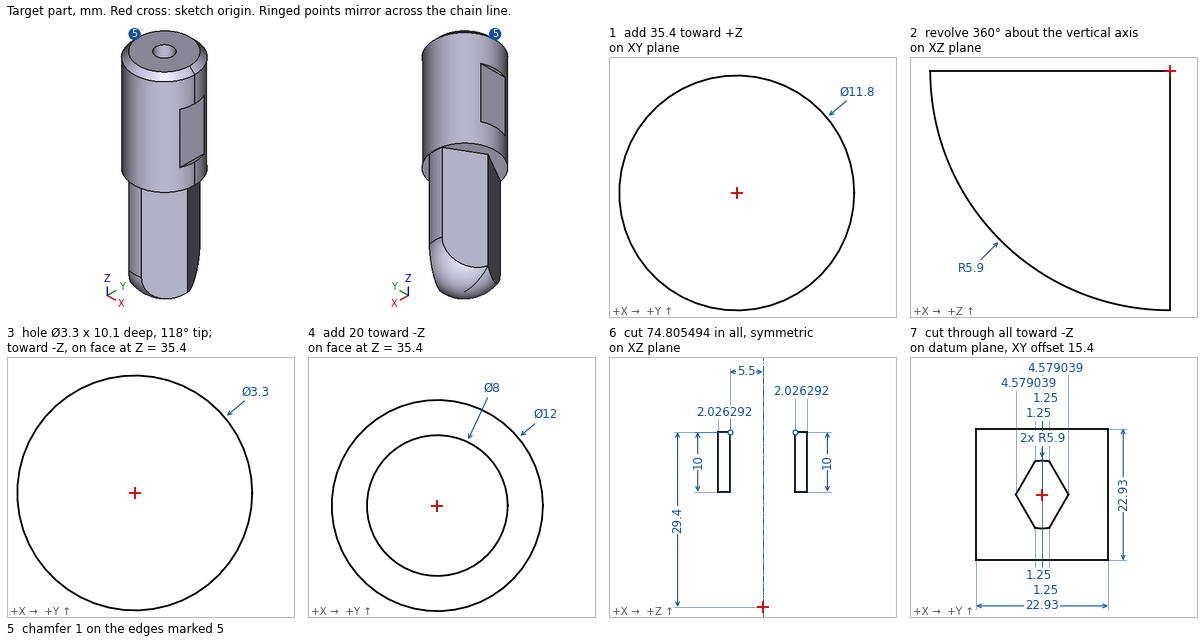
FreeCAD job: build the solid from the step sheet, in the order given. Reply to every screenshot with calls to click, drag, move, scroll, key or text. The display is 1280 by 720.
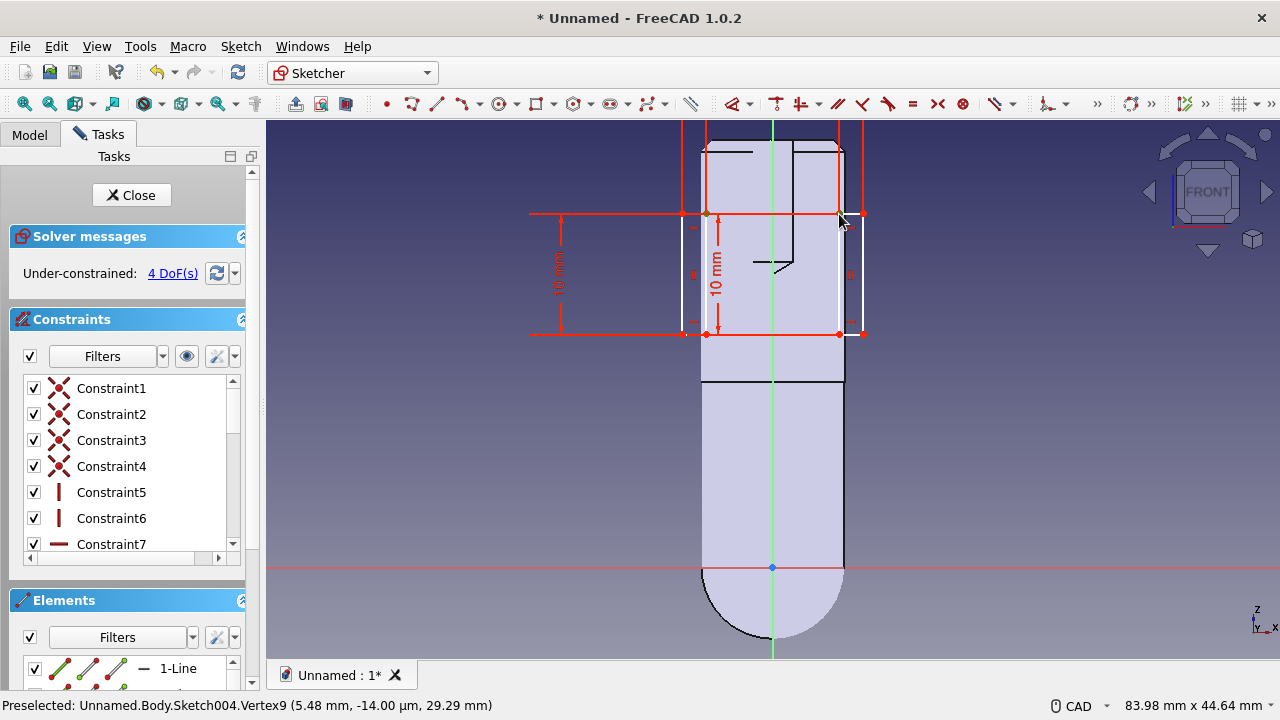
click(773, 528)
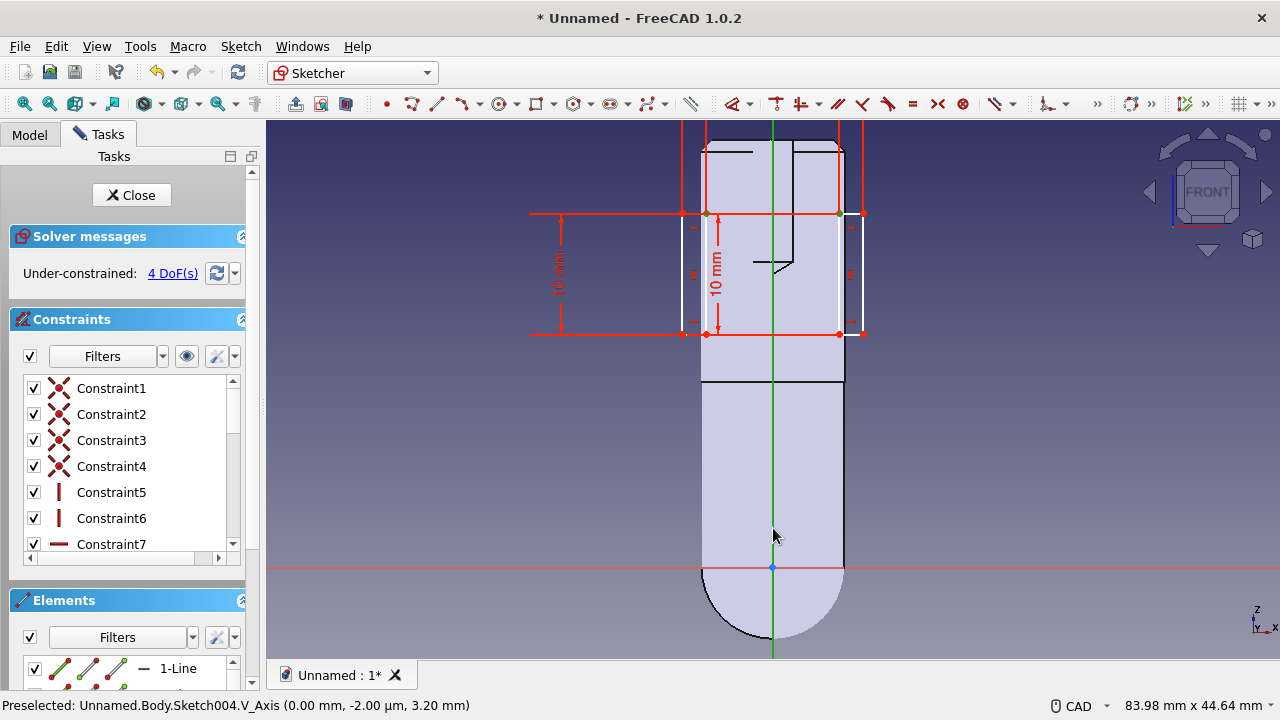
click(938, 104)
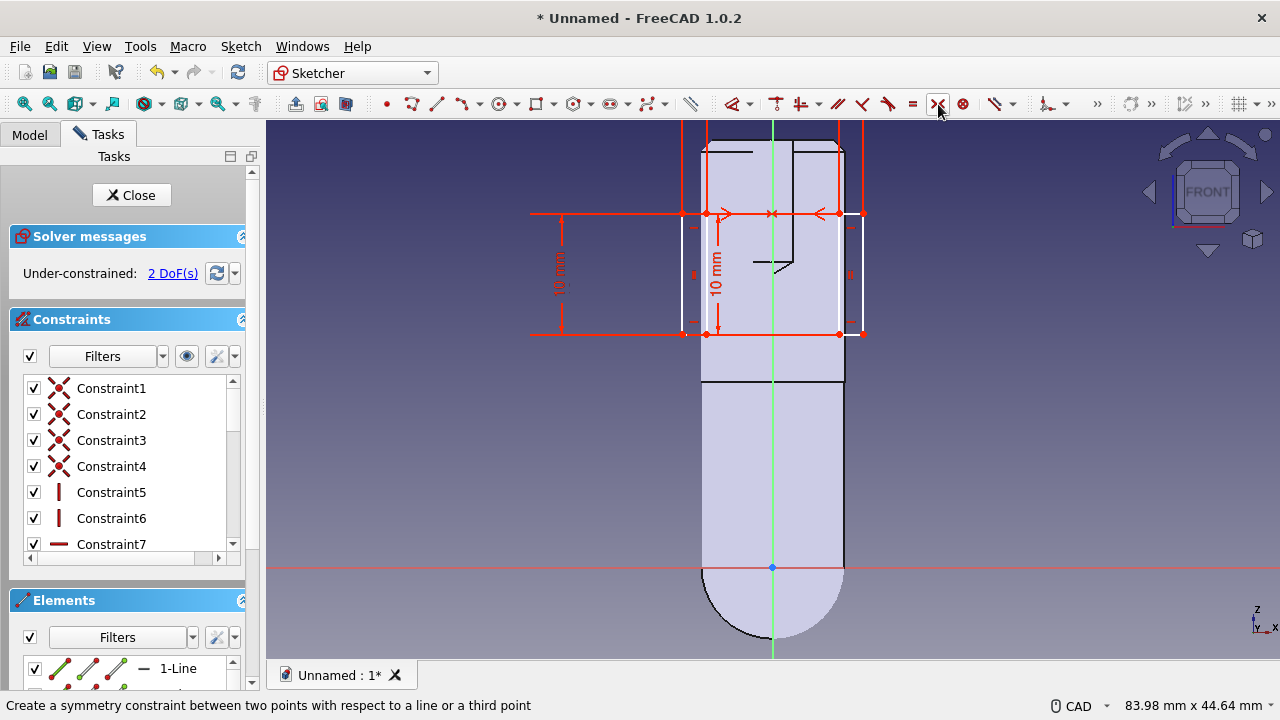
key(d)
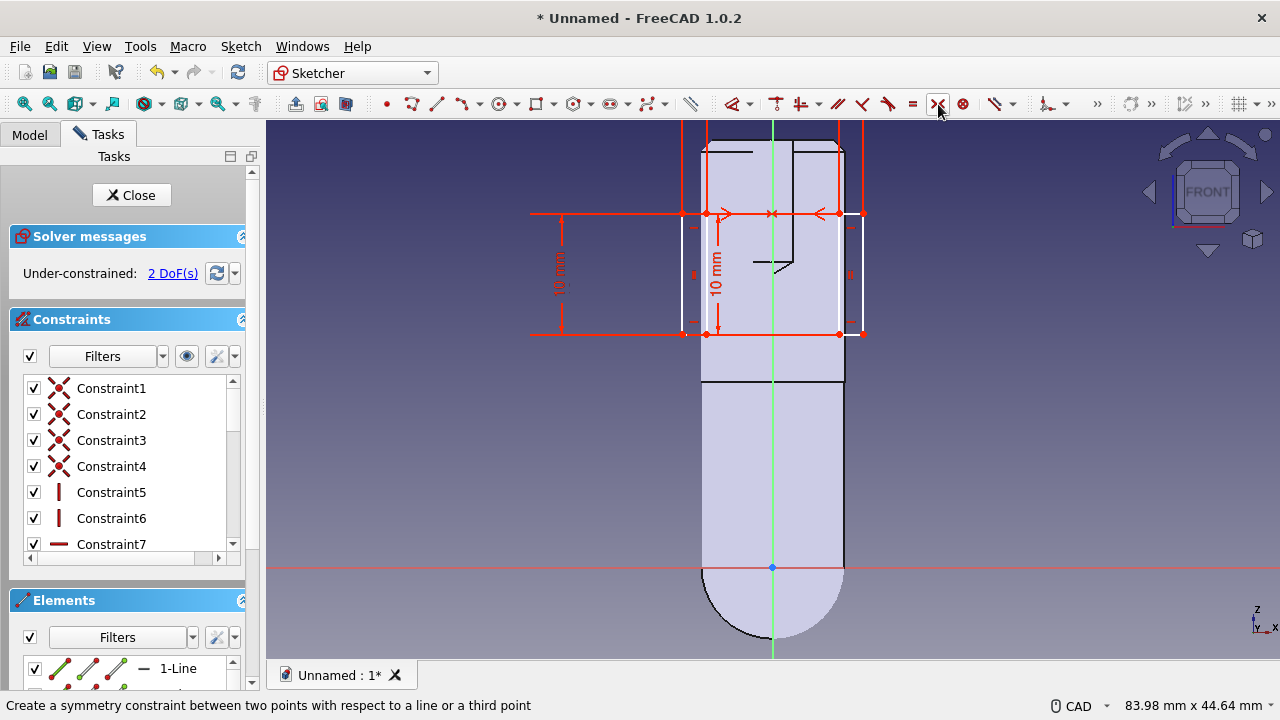
click(707, 335)
click(740, 602)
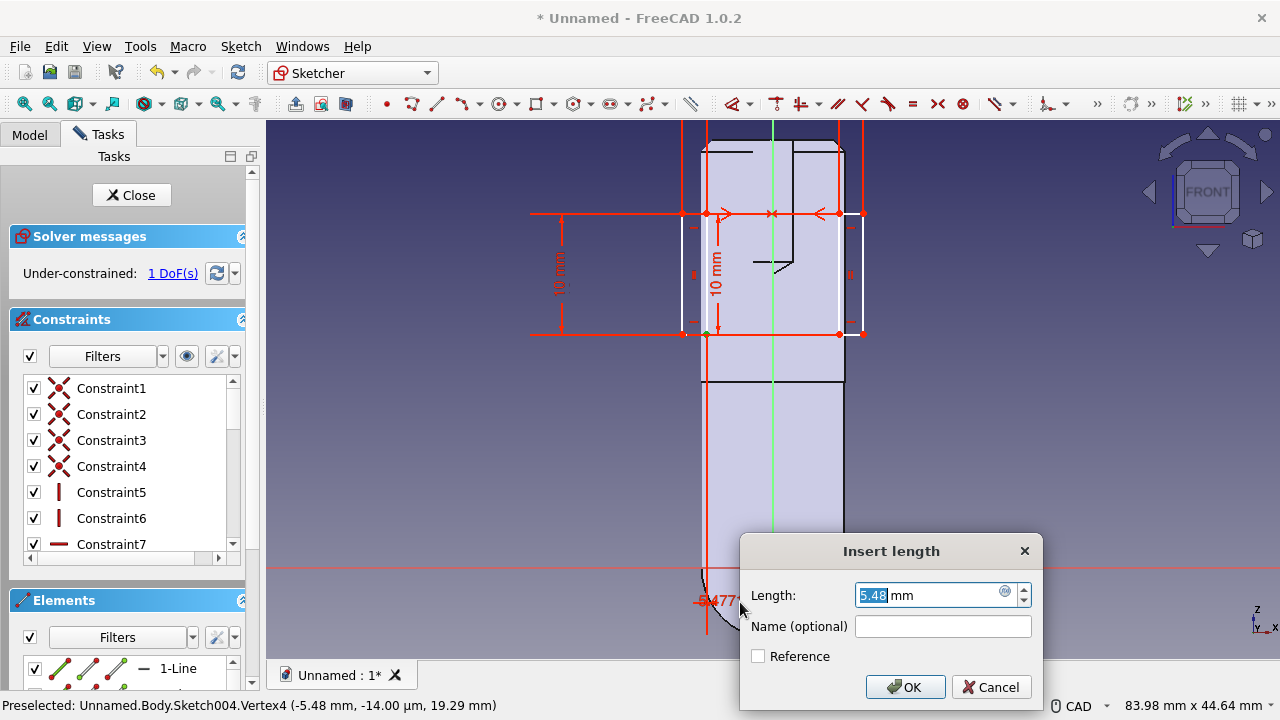
text(5.5)
key(Return)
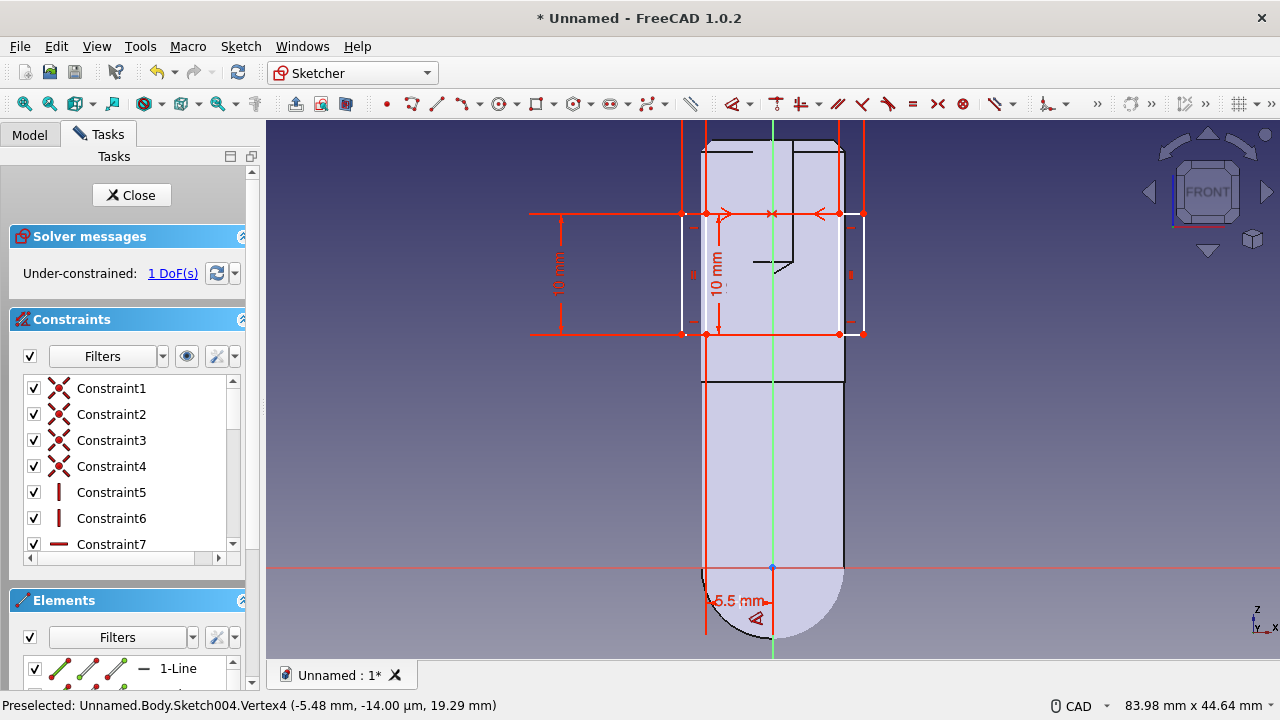
click(682, 214)
click(648, 391)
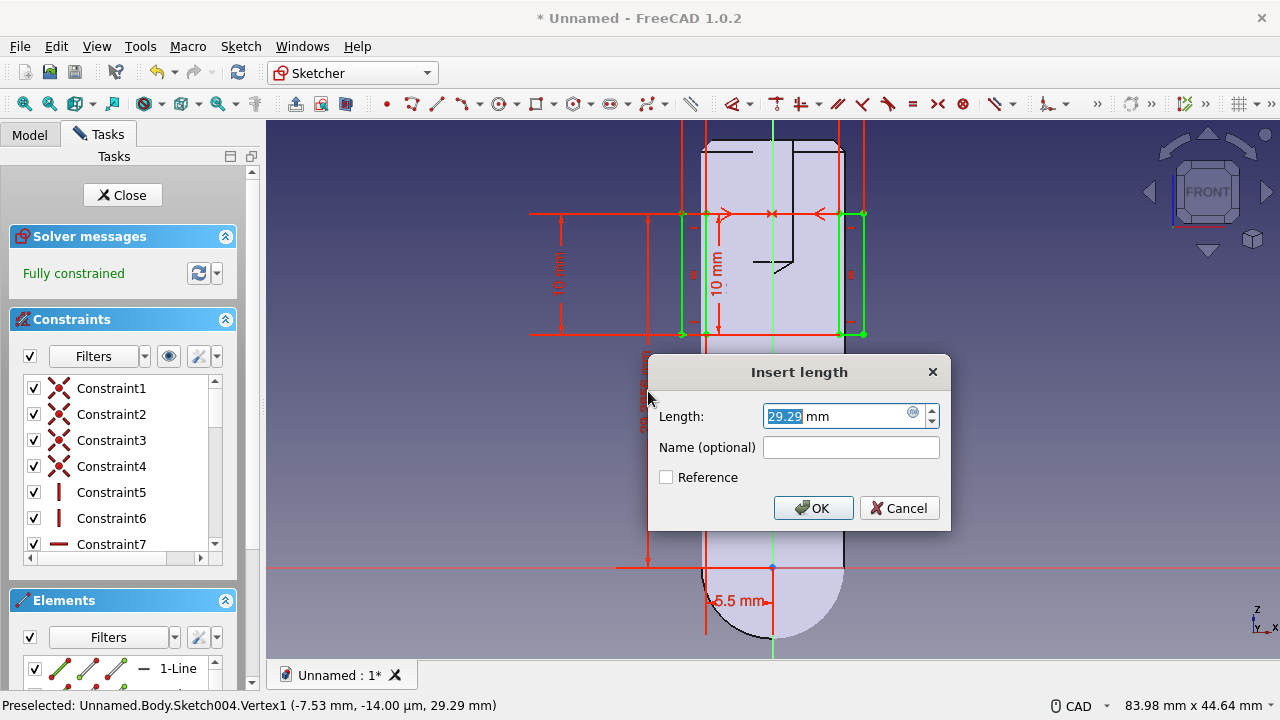
text(29.4)
key(Return)
key(Escape)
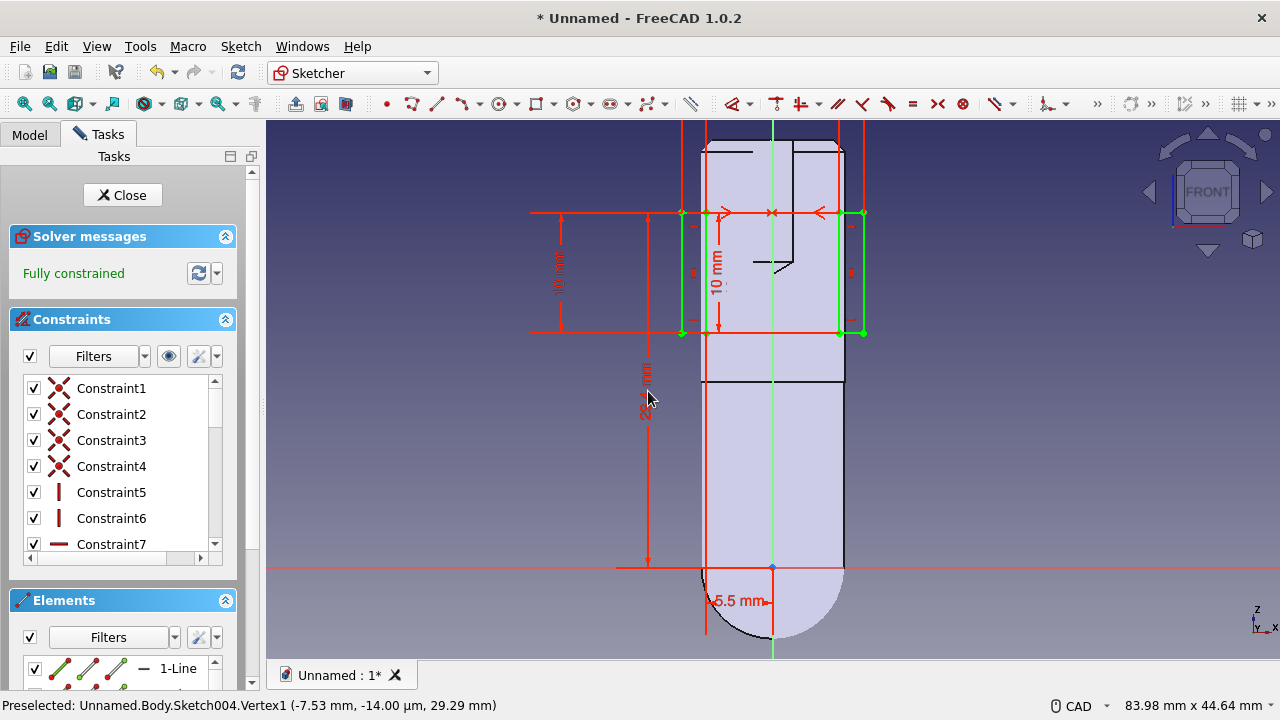
click(123, 195)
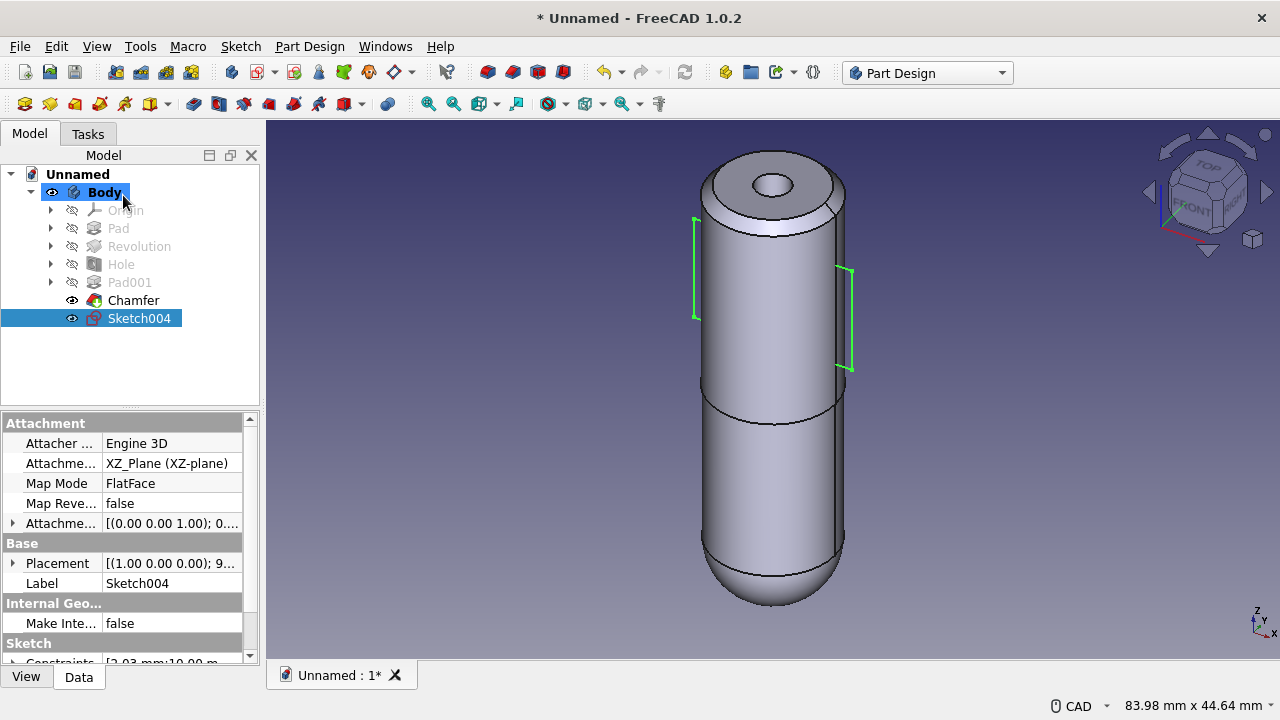
click(194, 104)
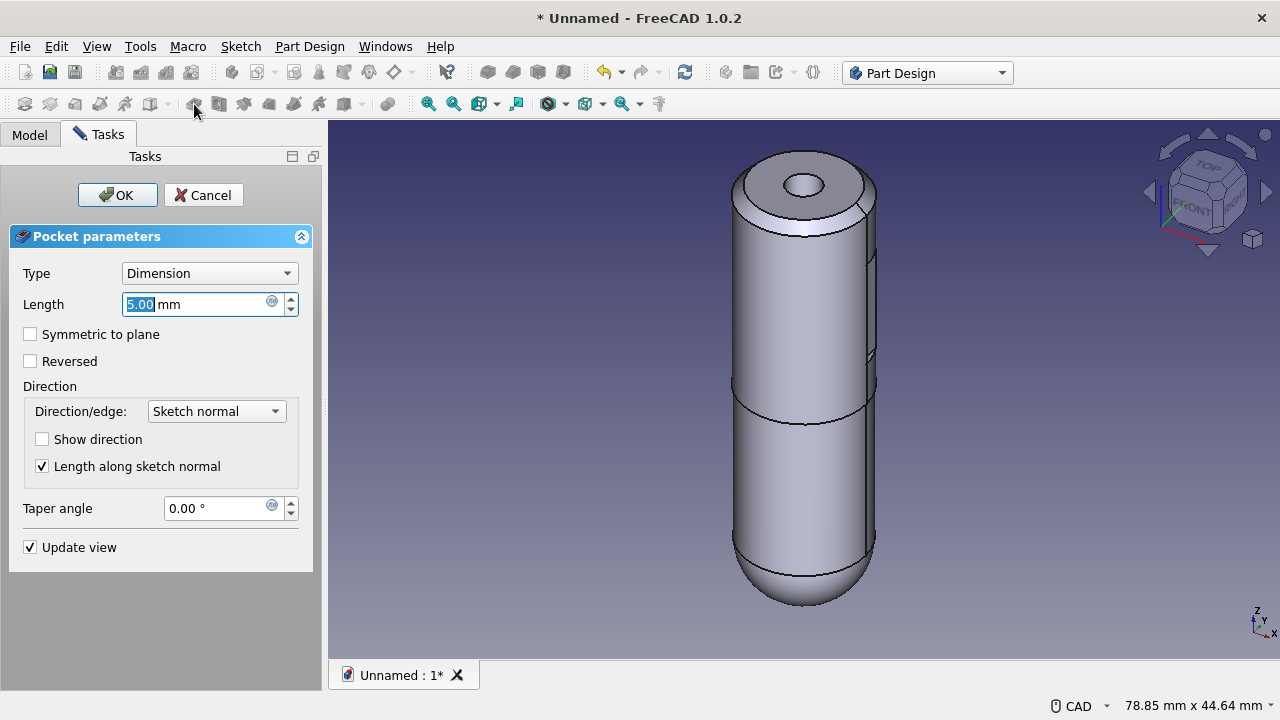
text(74.805494)
key(Tab)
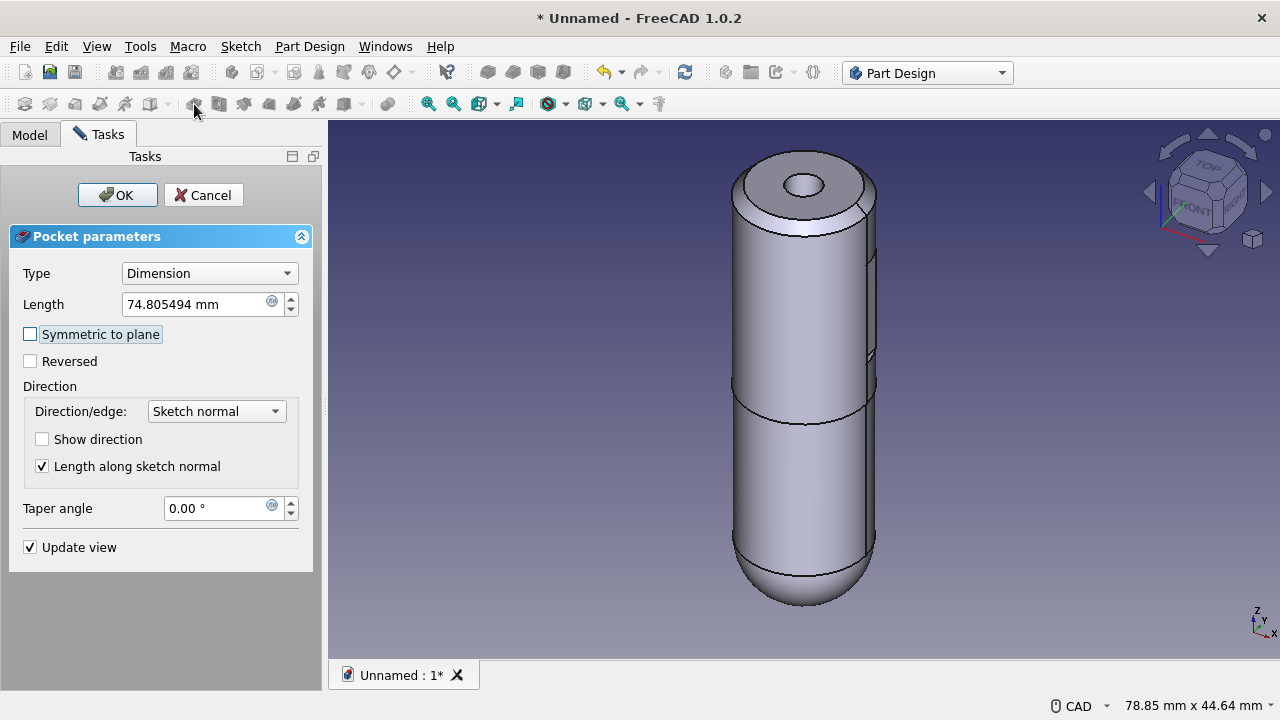
click(31, 334)